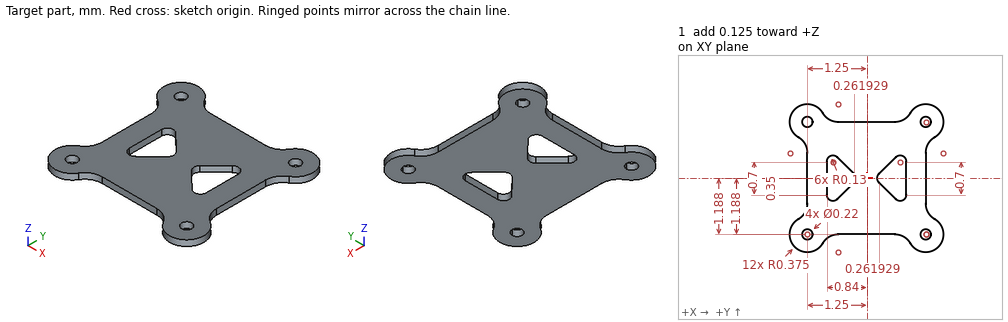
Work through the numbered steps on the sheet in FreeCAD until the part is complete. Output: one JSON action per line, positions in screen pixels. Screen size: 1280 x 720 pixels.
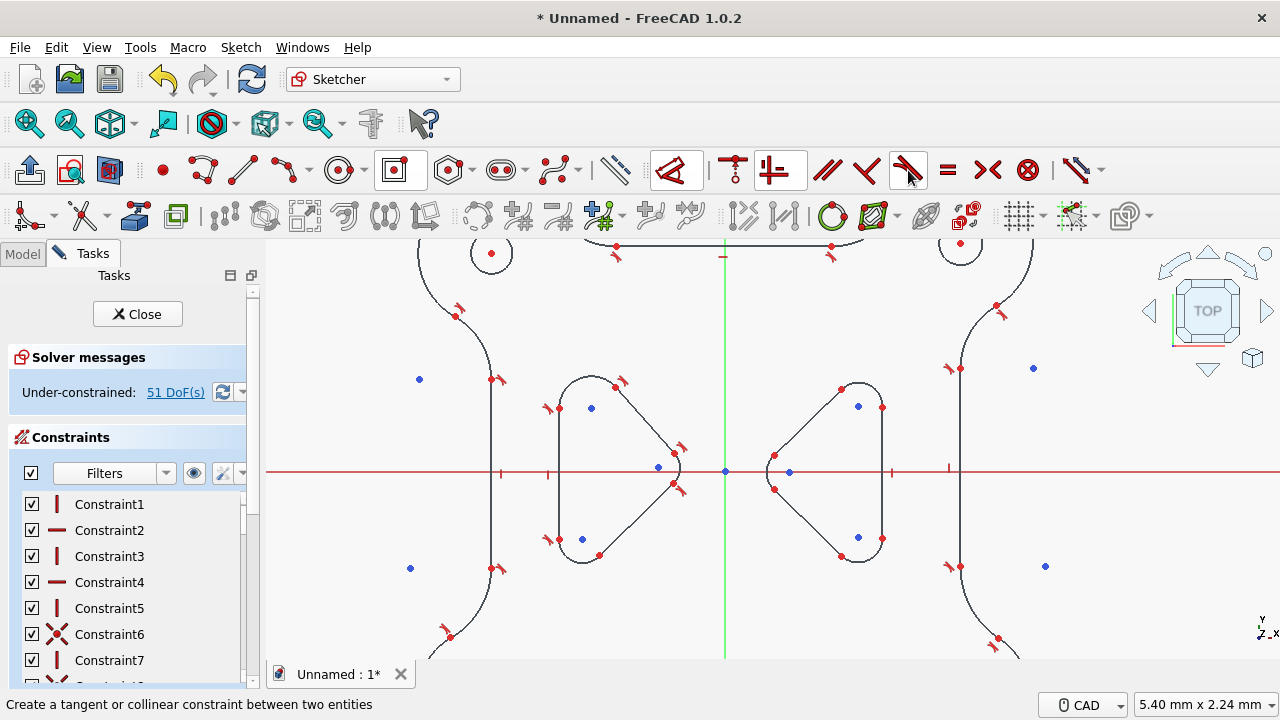
{"action": "left_click", "coordinate": [651, 505]}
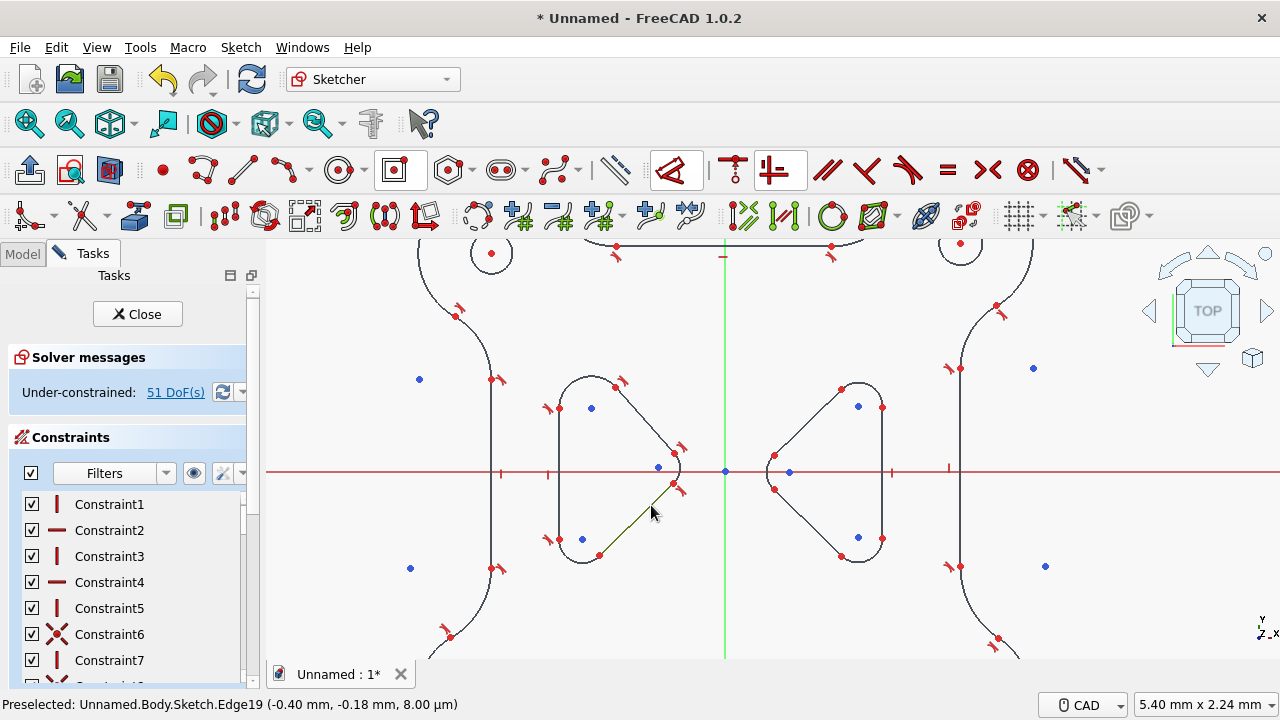
{"action": "left_click", "coordinate": [565, 555]}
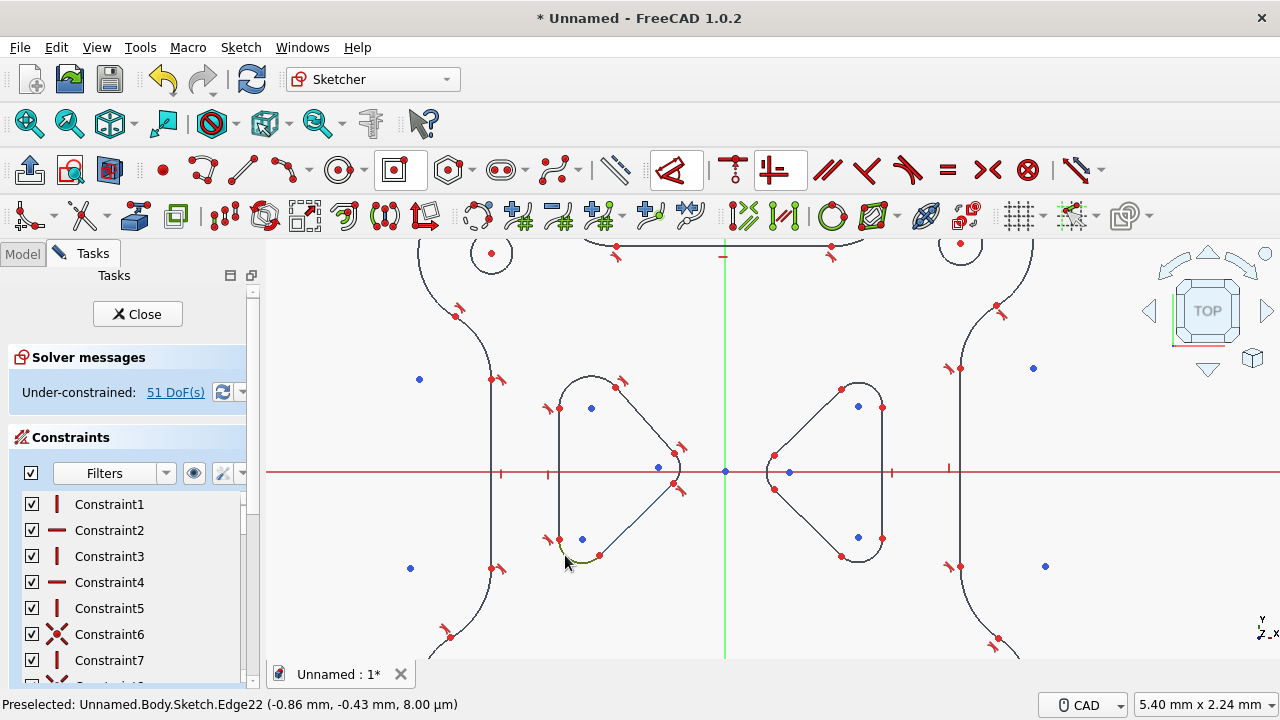
{"action": "left_click", "coordinate": [908, 170]}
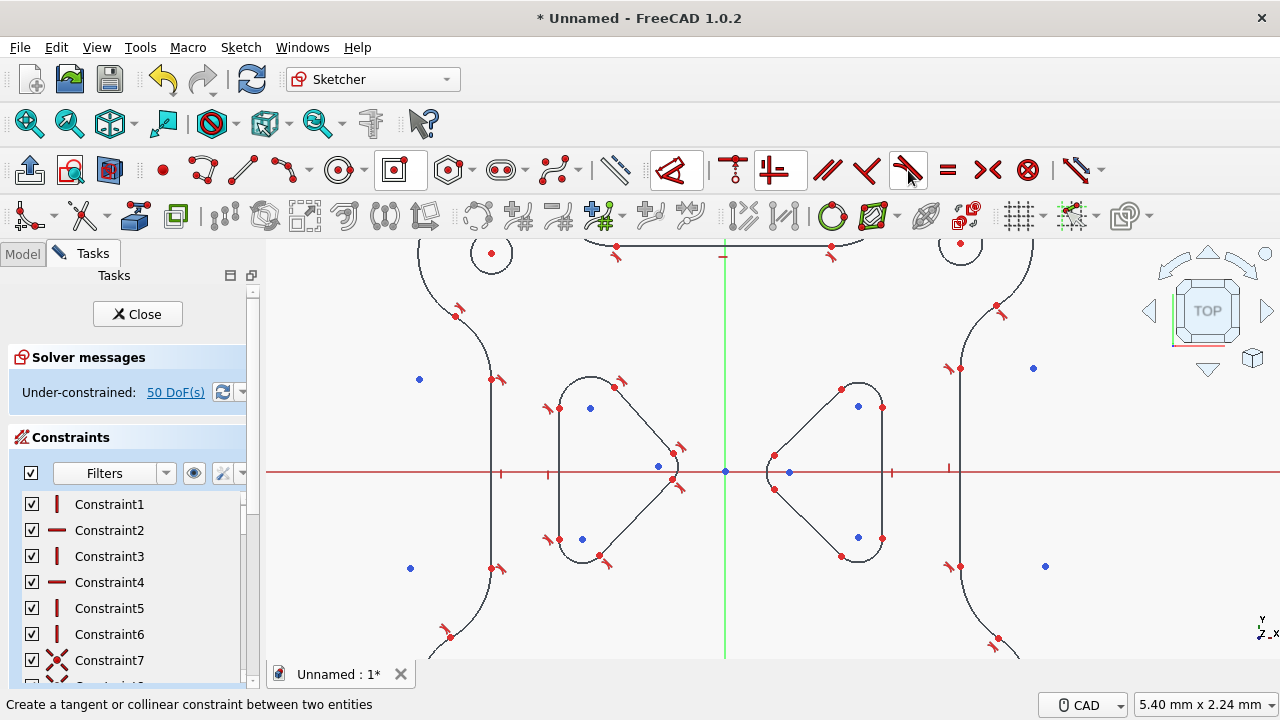
{"action": "left_click", "coordinate": [821, 536]}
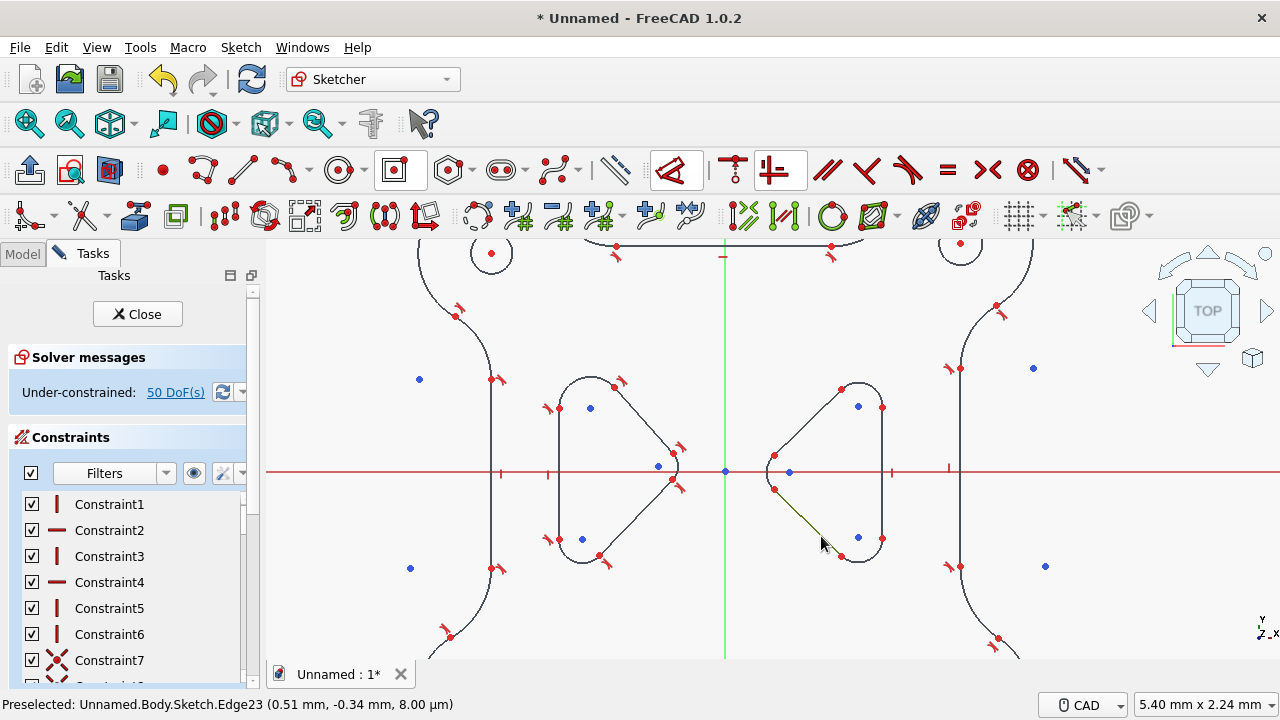
{"action": "left_click", "coordinate": [767, 473]}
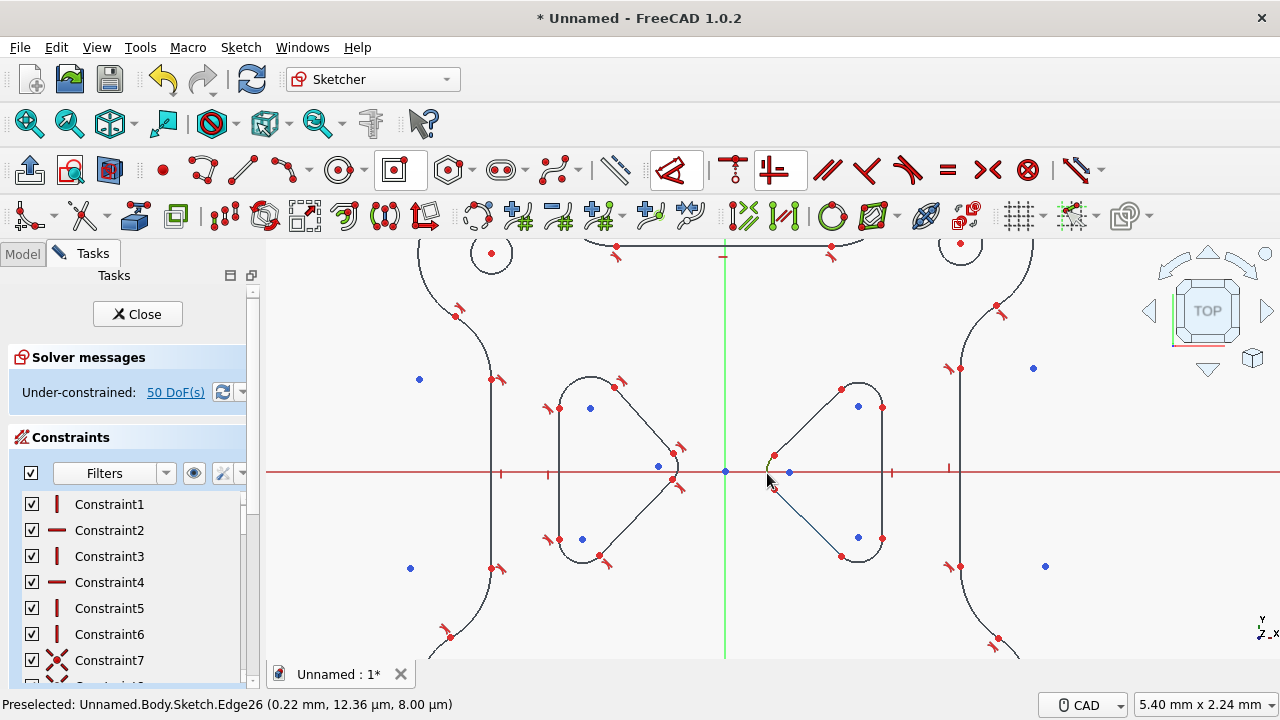
{"action": "left_click", "coordinate": [908, 170]}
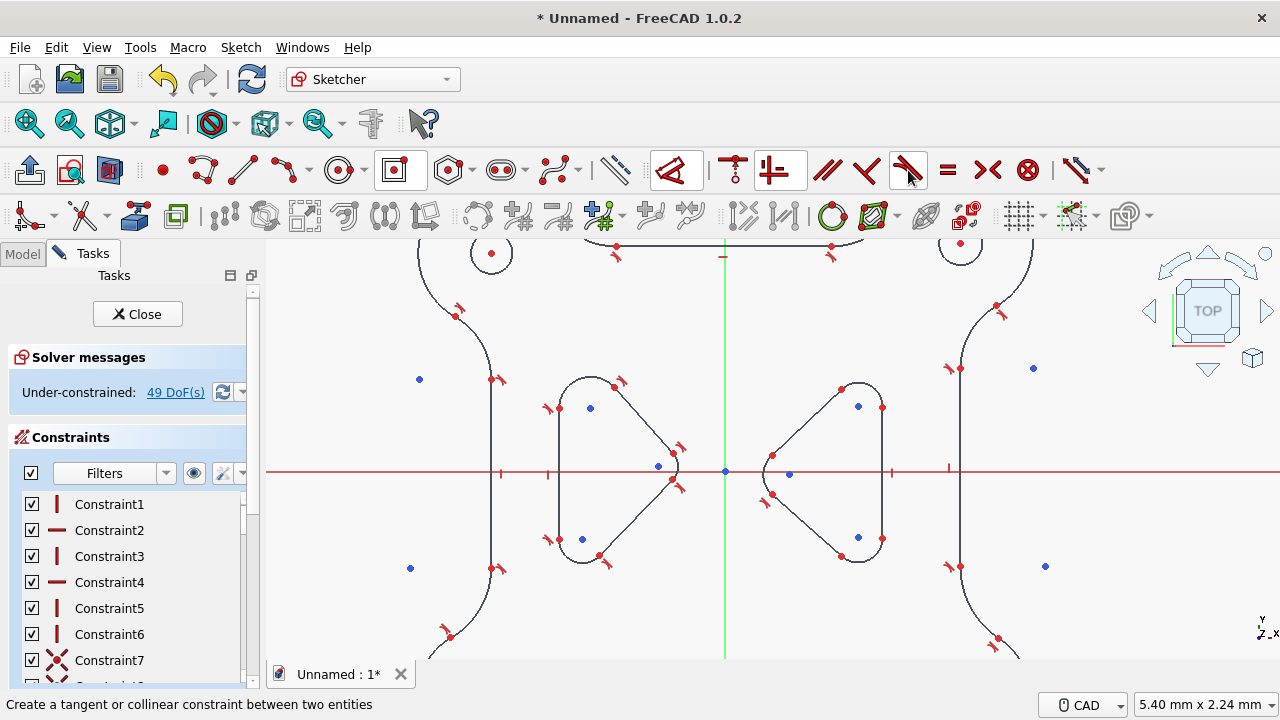
{"action": "left_click", "coordinate": [821, 538]}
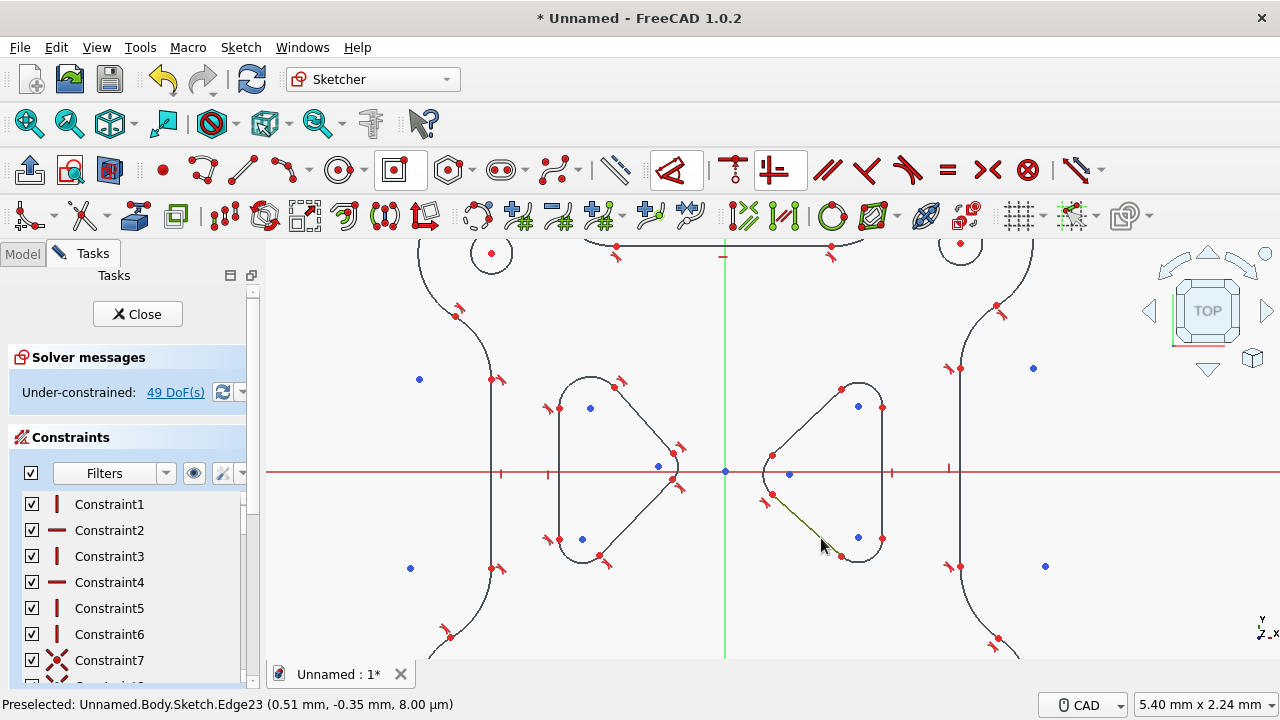
{"action": "left_click", "coordinate": [857, 562]}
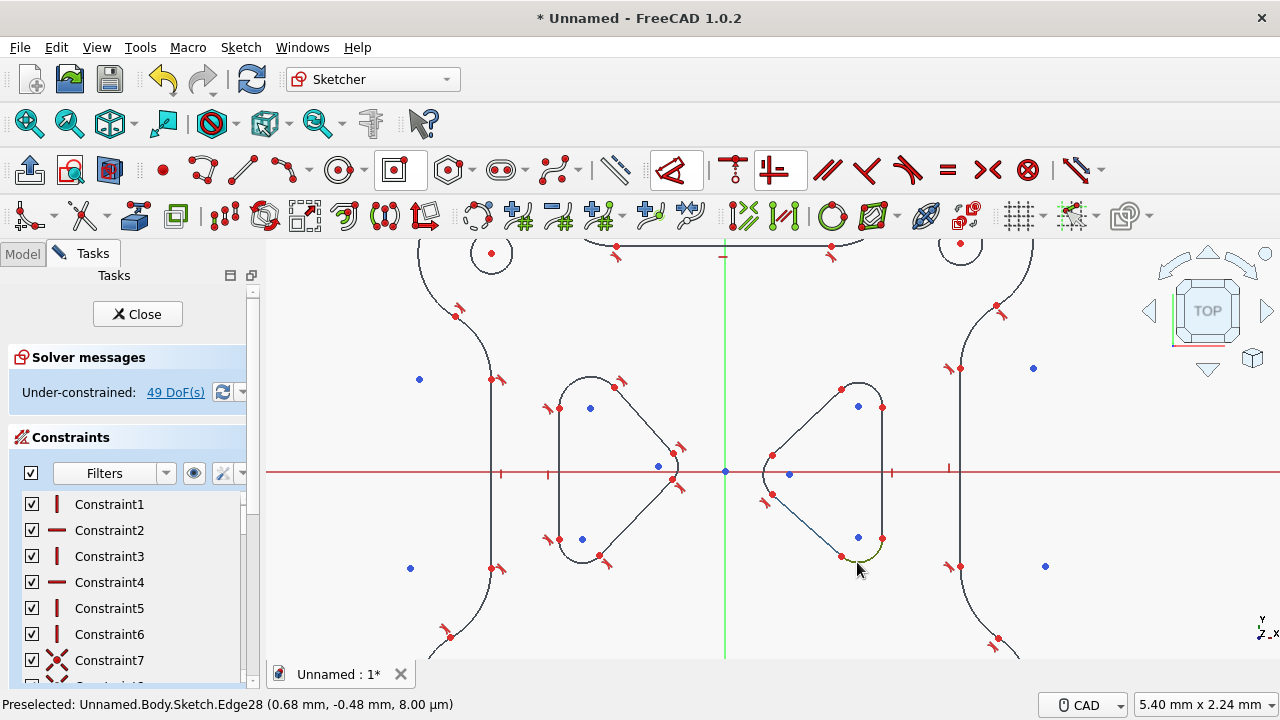
{"action": "left_click", "coordinate": [908, 170]}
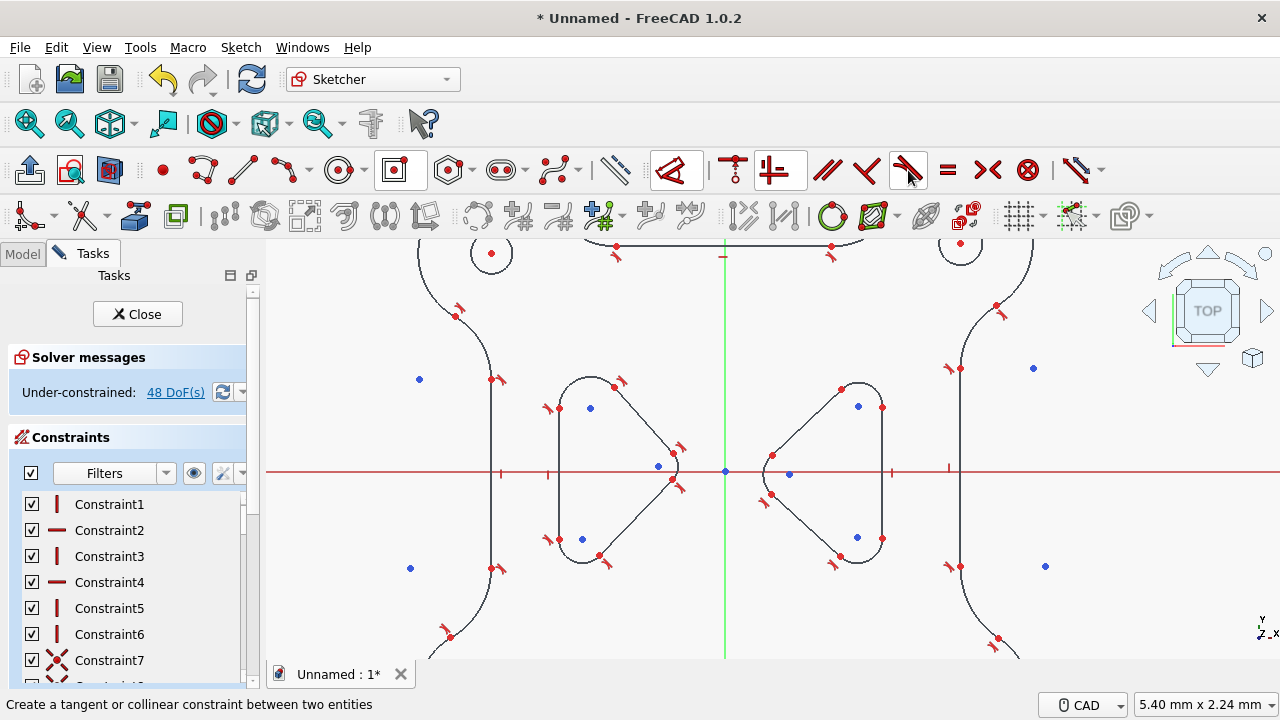
{"action": "left_click", "coordinate": [793, 436]}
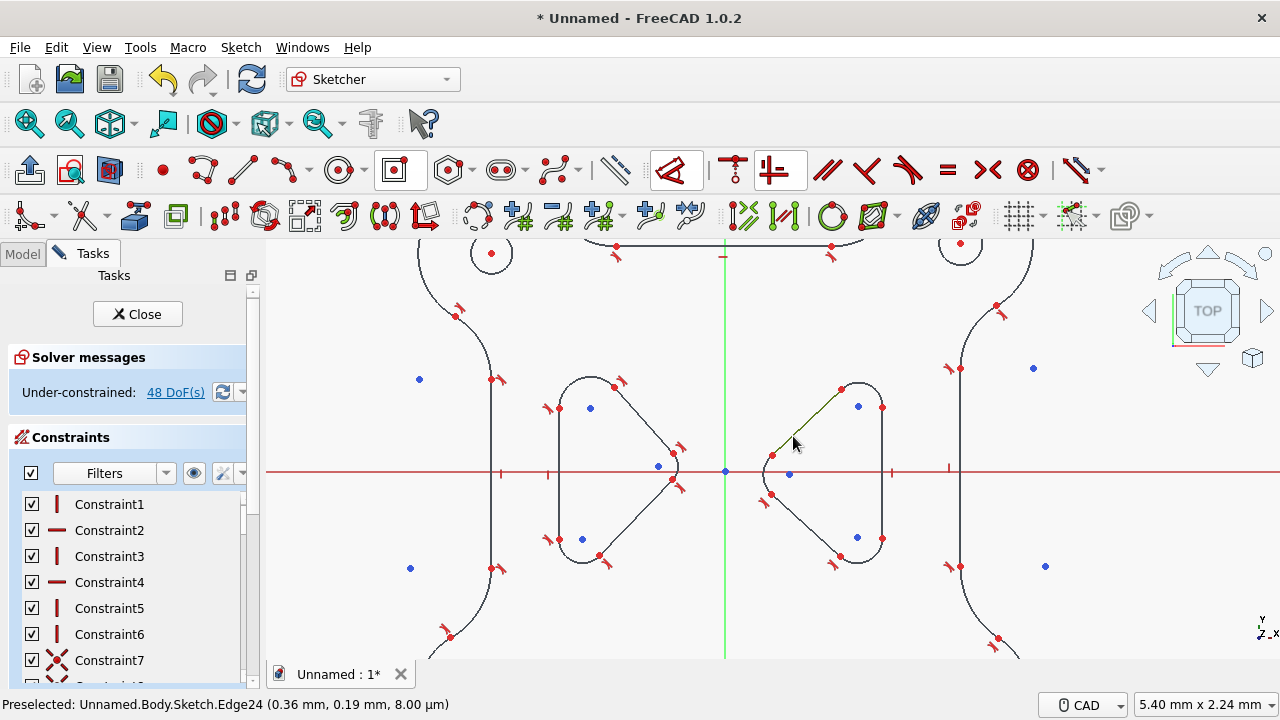
{"action": "left_click", "coordinate": [765, 483]}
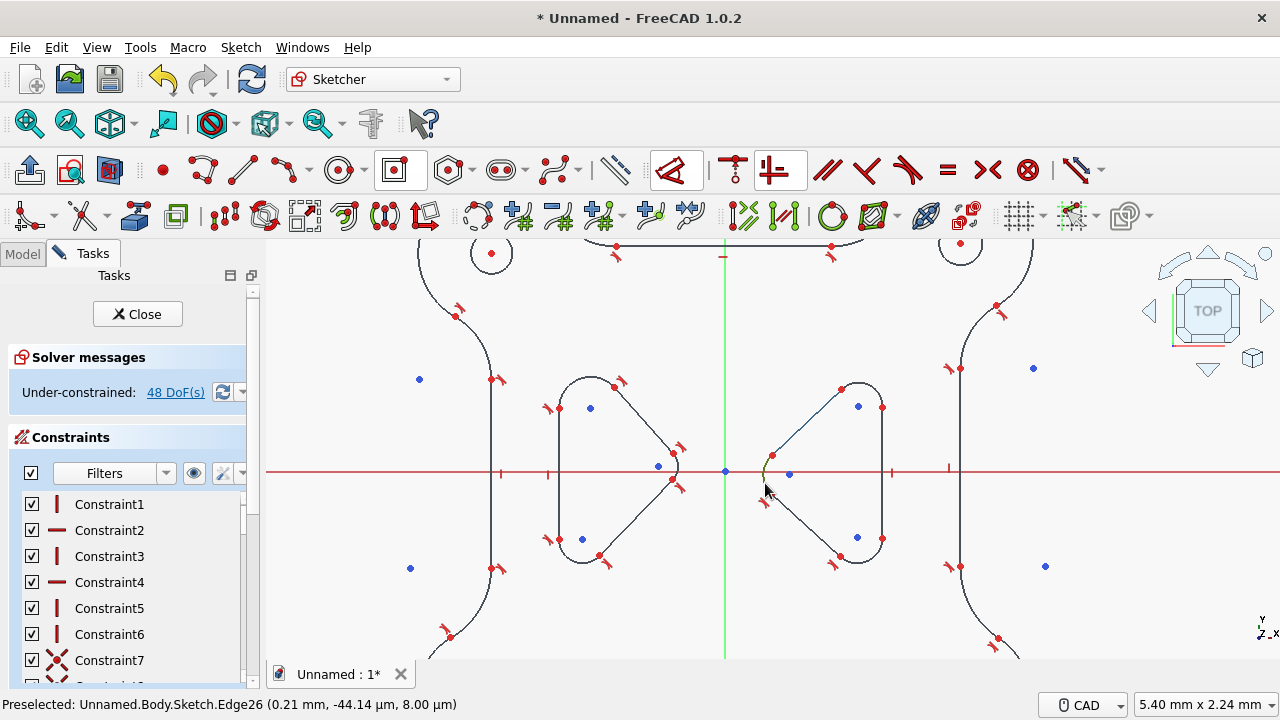
{"action": "left_click", "coordinate": [908, 170]}